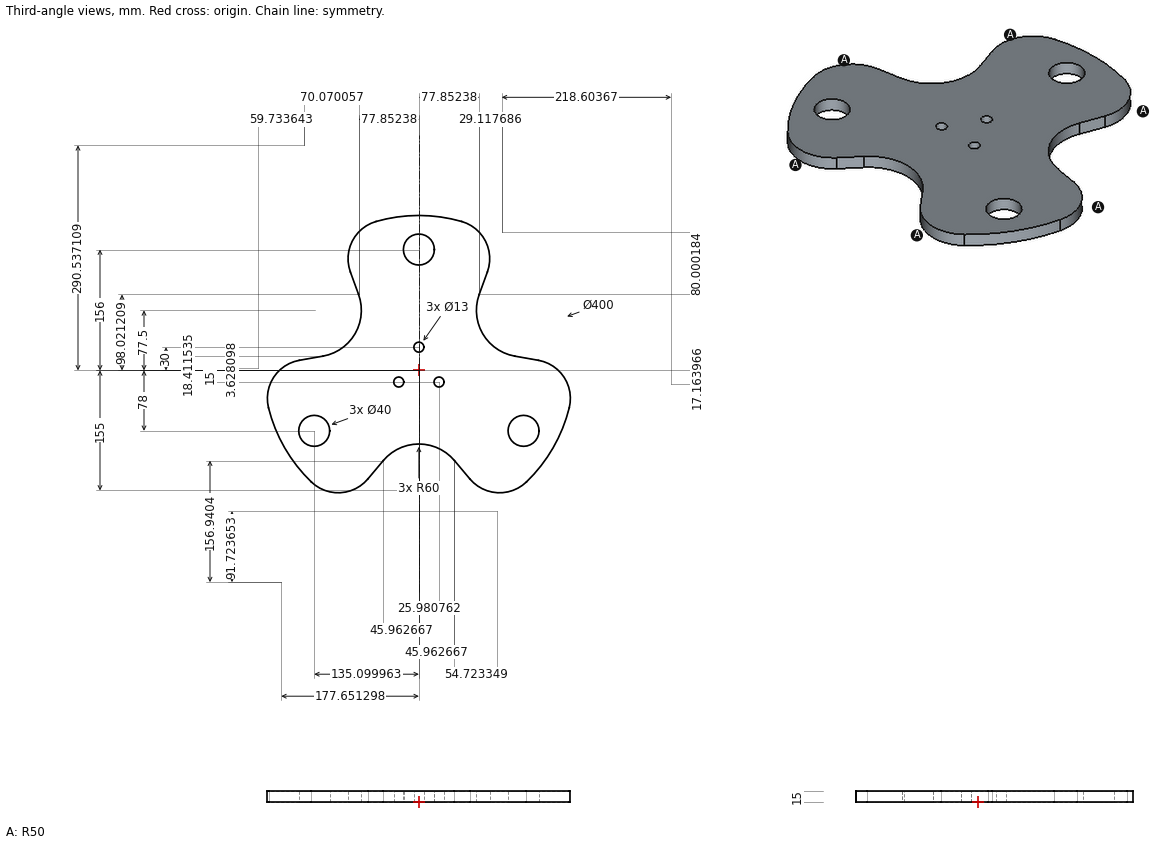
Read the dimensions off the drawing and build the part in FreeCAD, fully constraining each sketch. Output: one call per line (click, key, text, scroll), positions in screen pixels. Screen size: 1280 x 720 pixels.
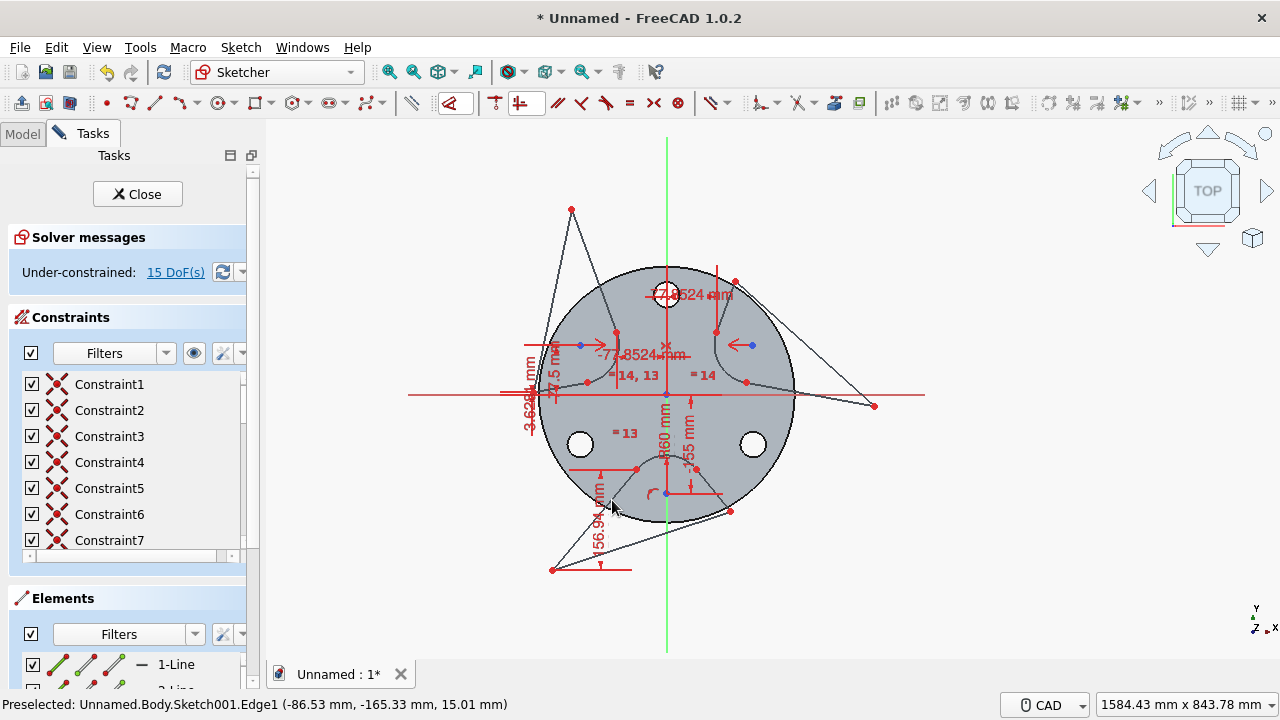
scroll(637, 470, up, 2)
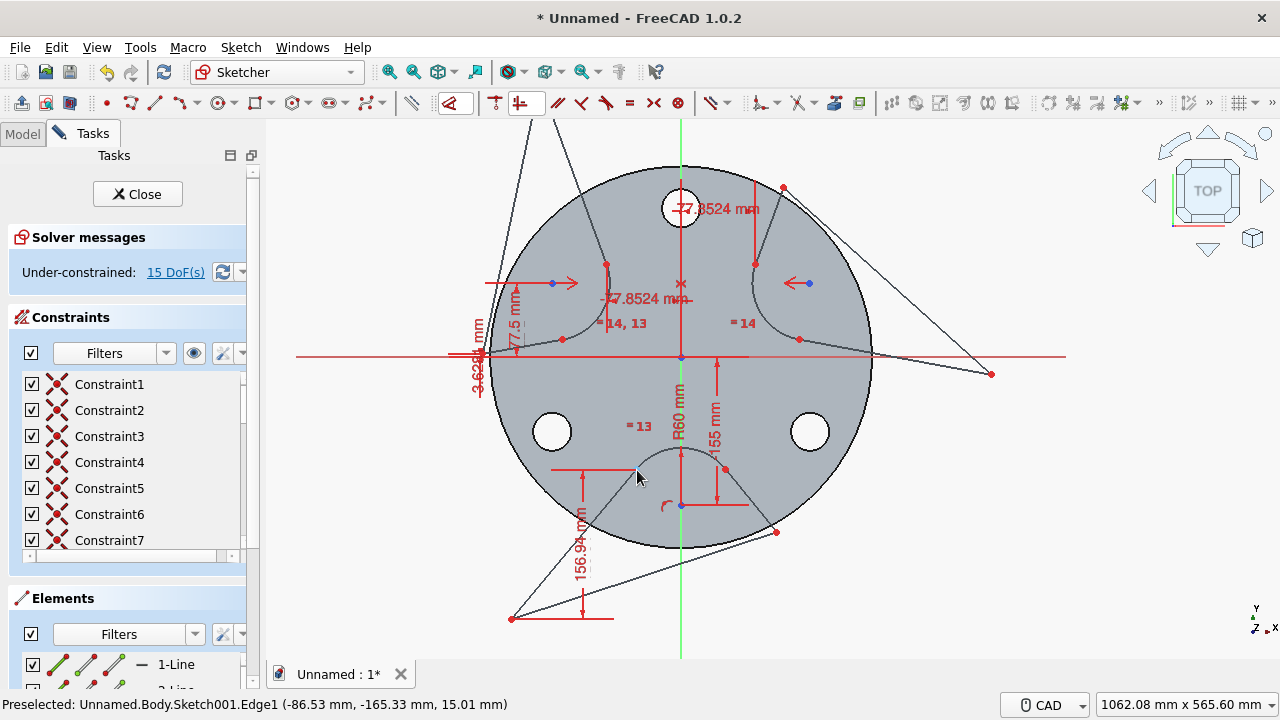
click(636, 470)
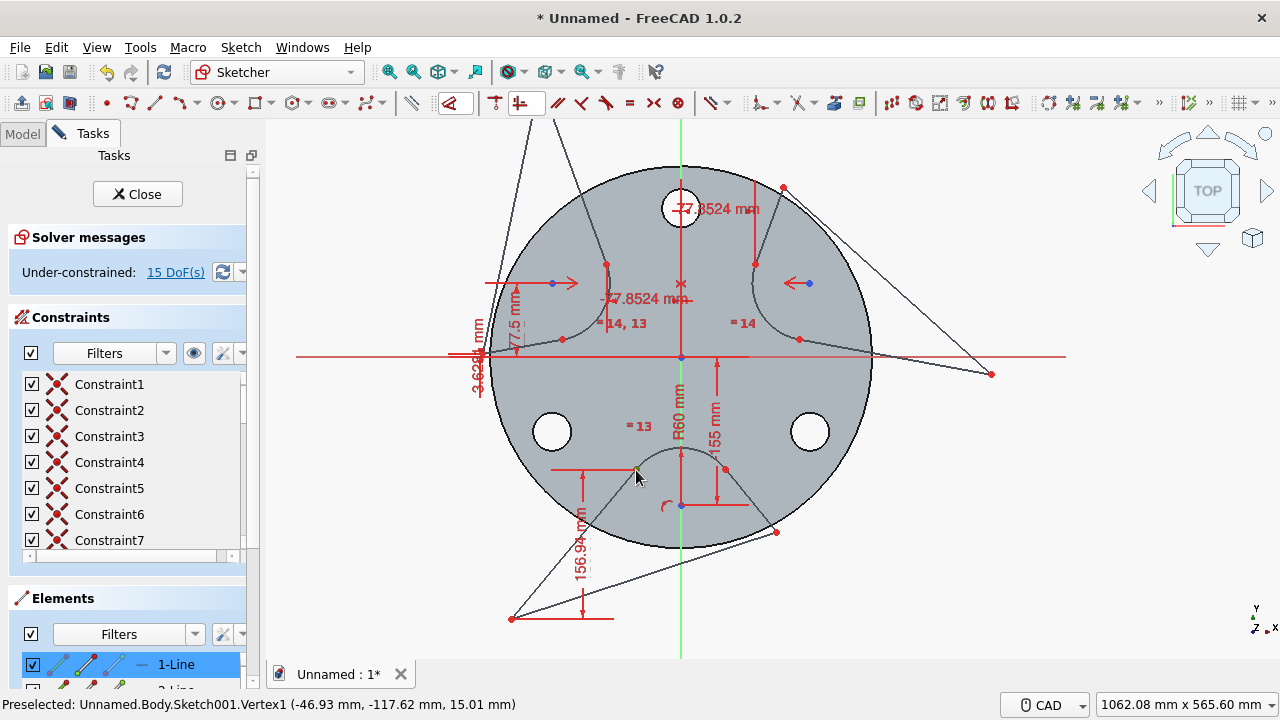
click(468, 104)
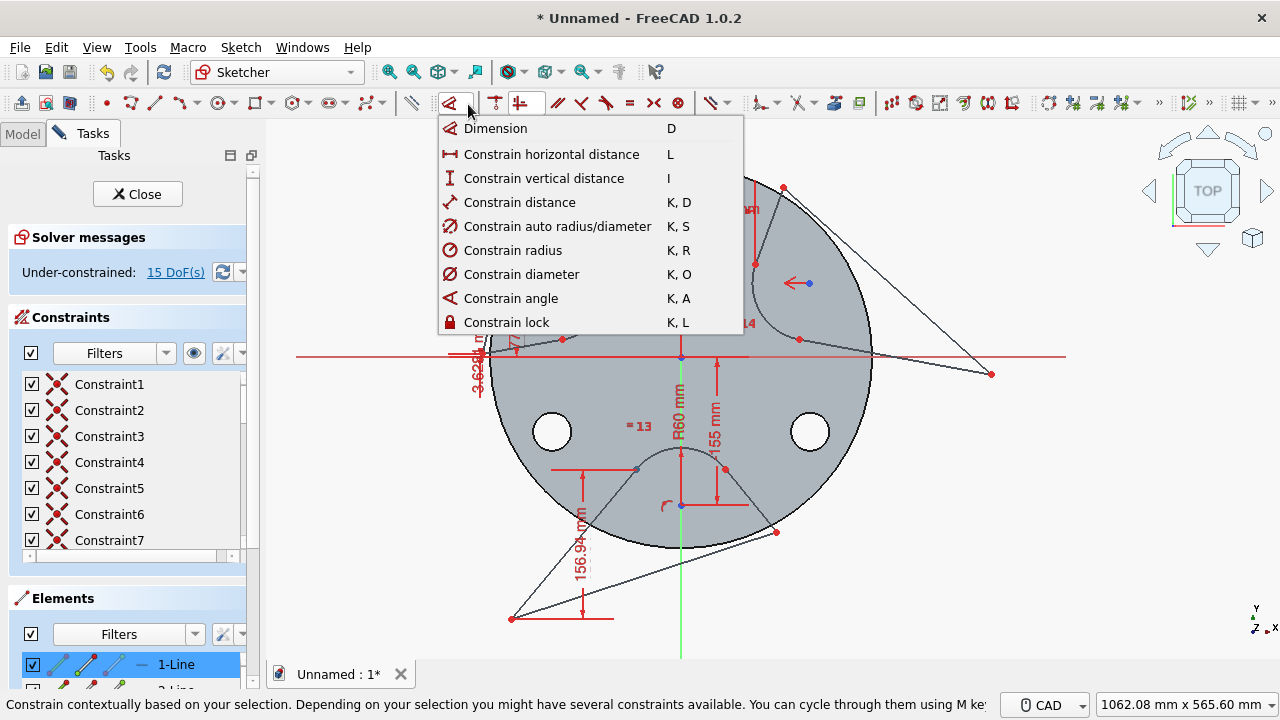
click(591, 154)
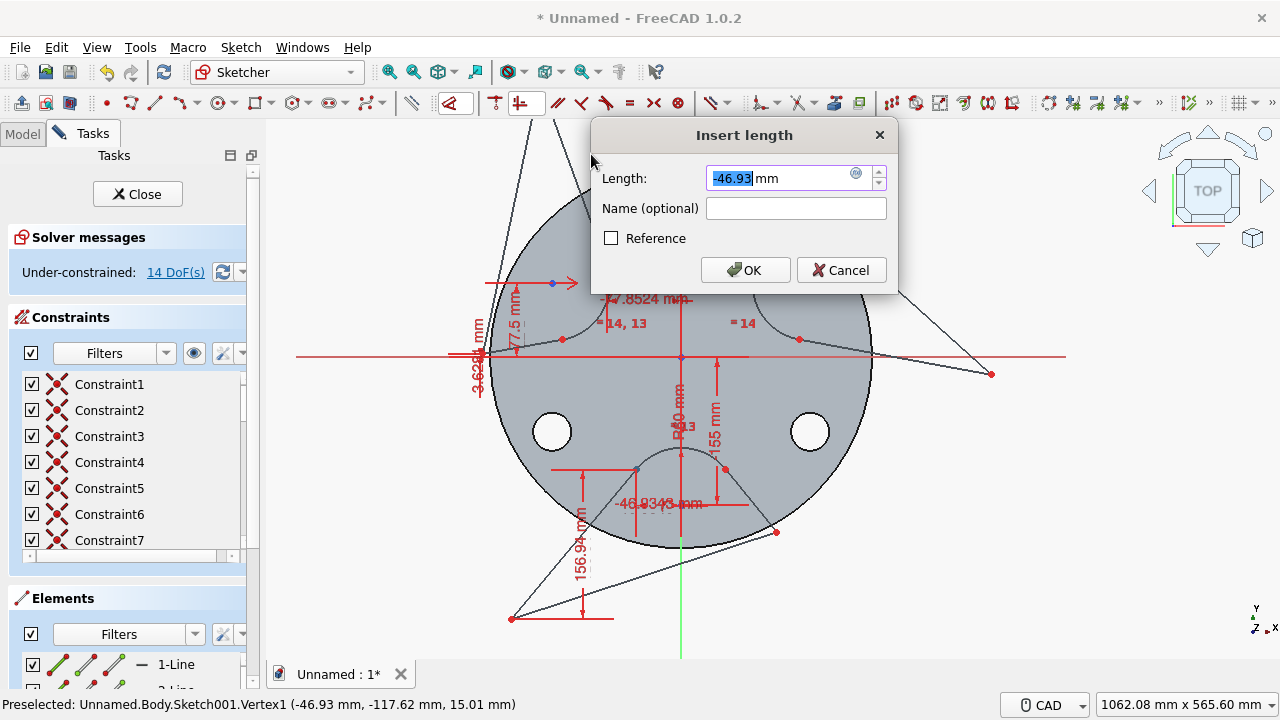
text(-45.962667)
key(Return)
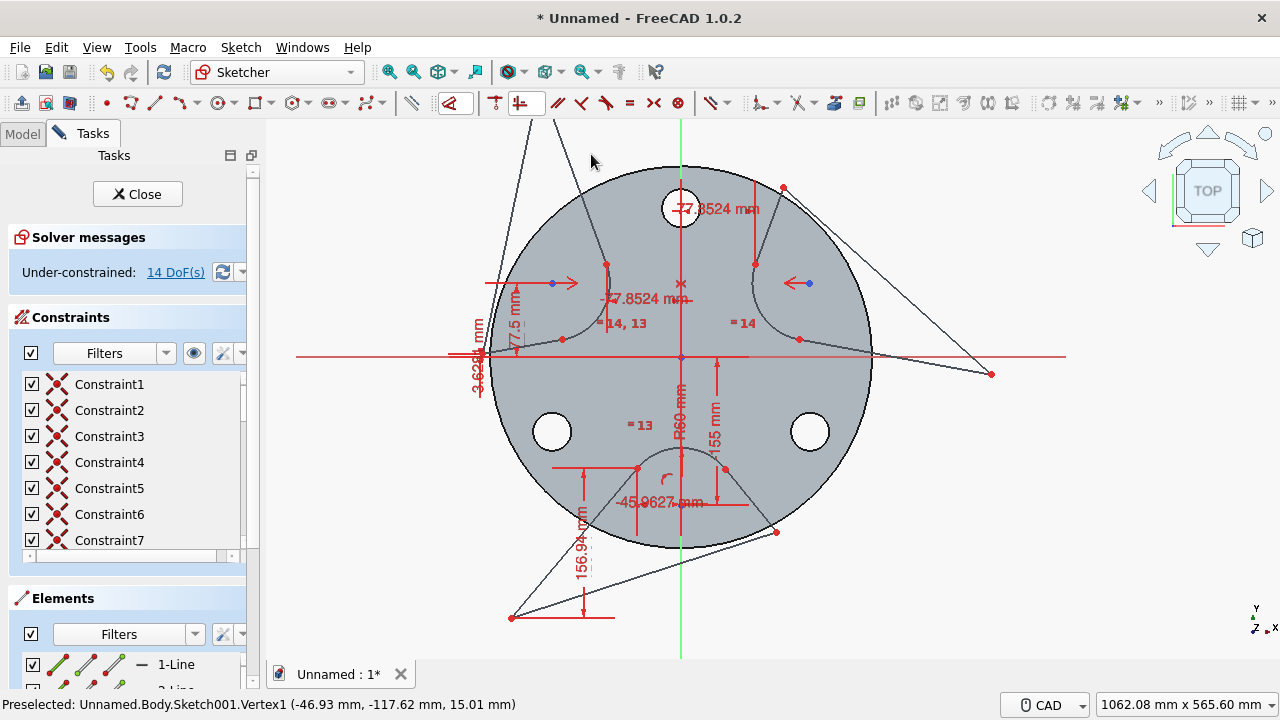
click(726, 469)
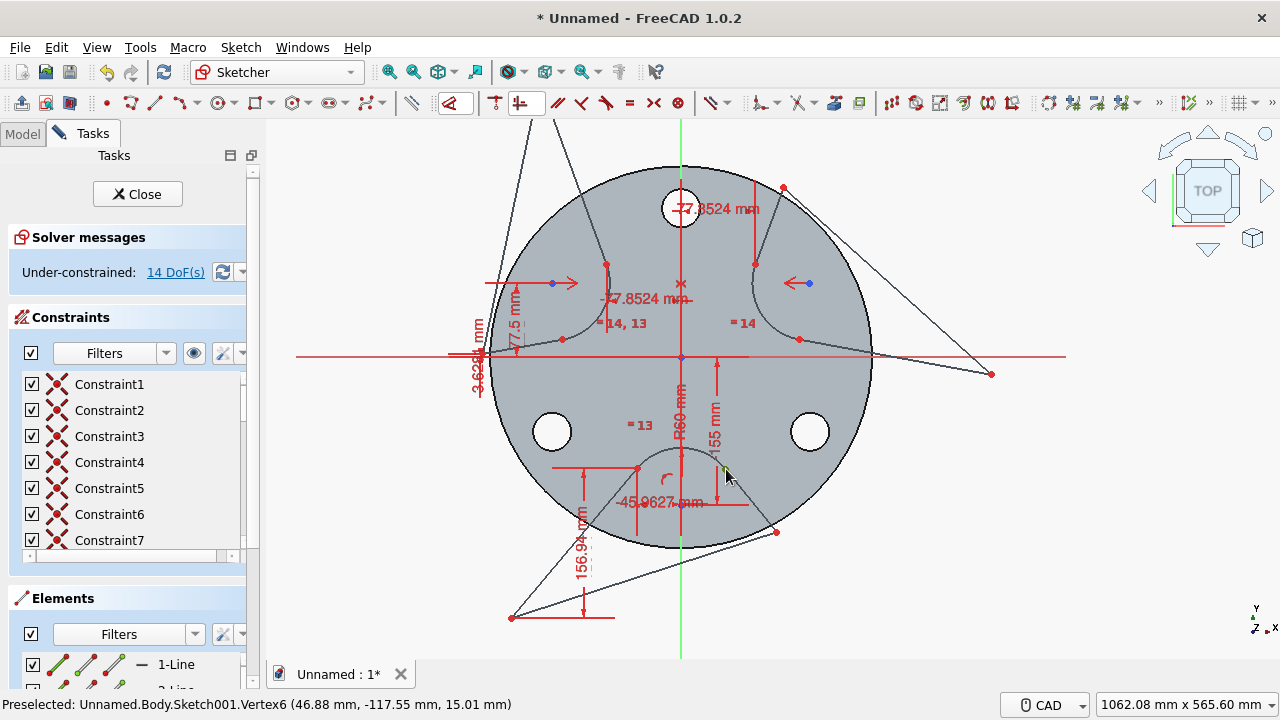
click(468, 104)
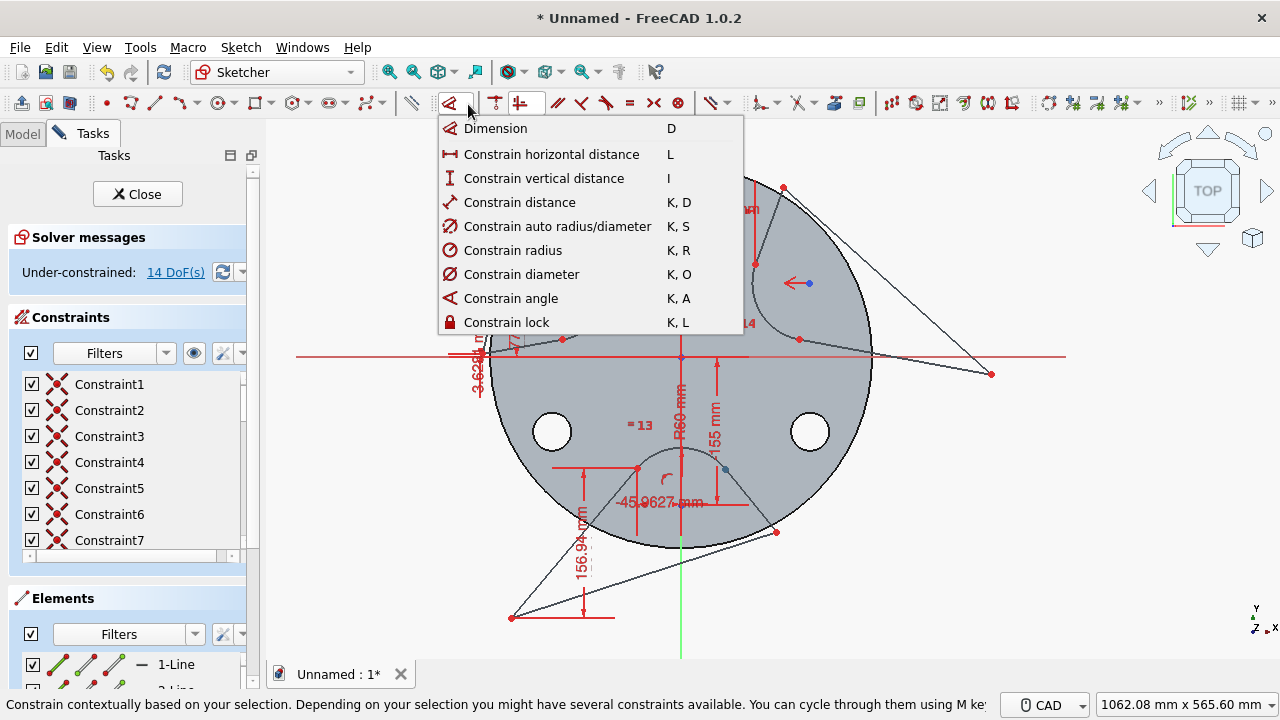
click(591, 154)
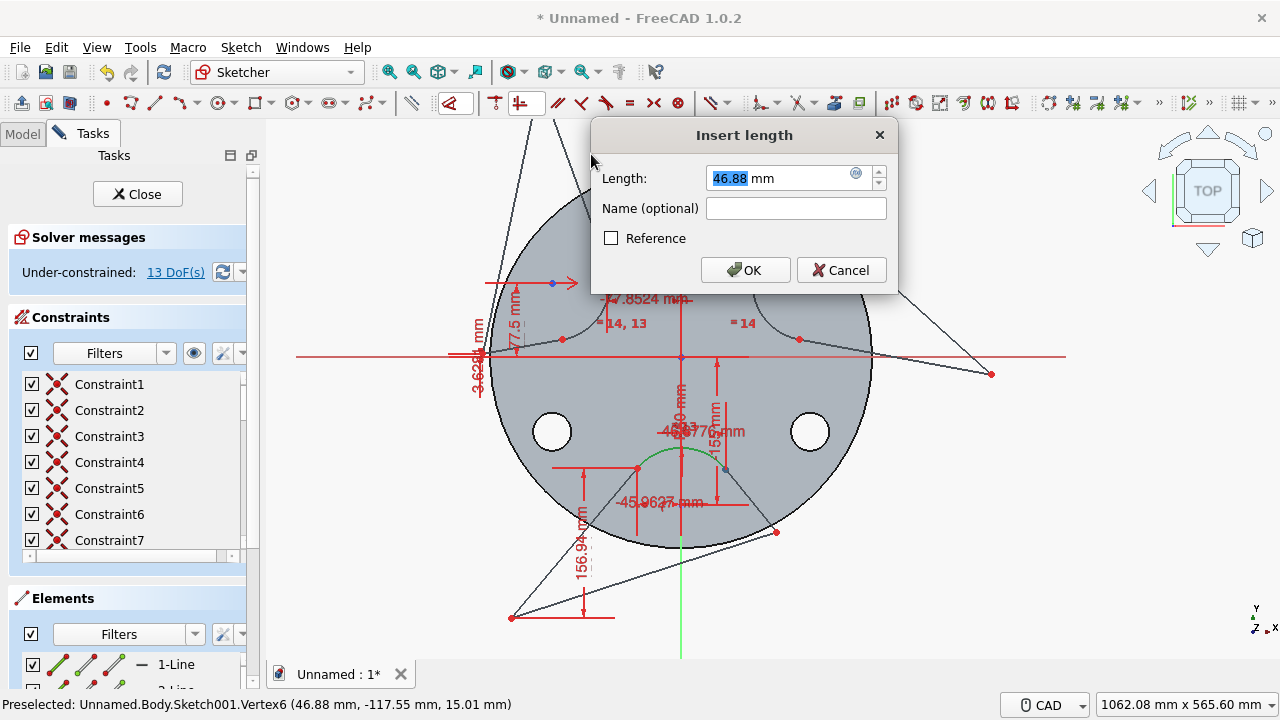
text(45.962667)
key(Return)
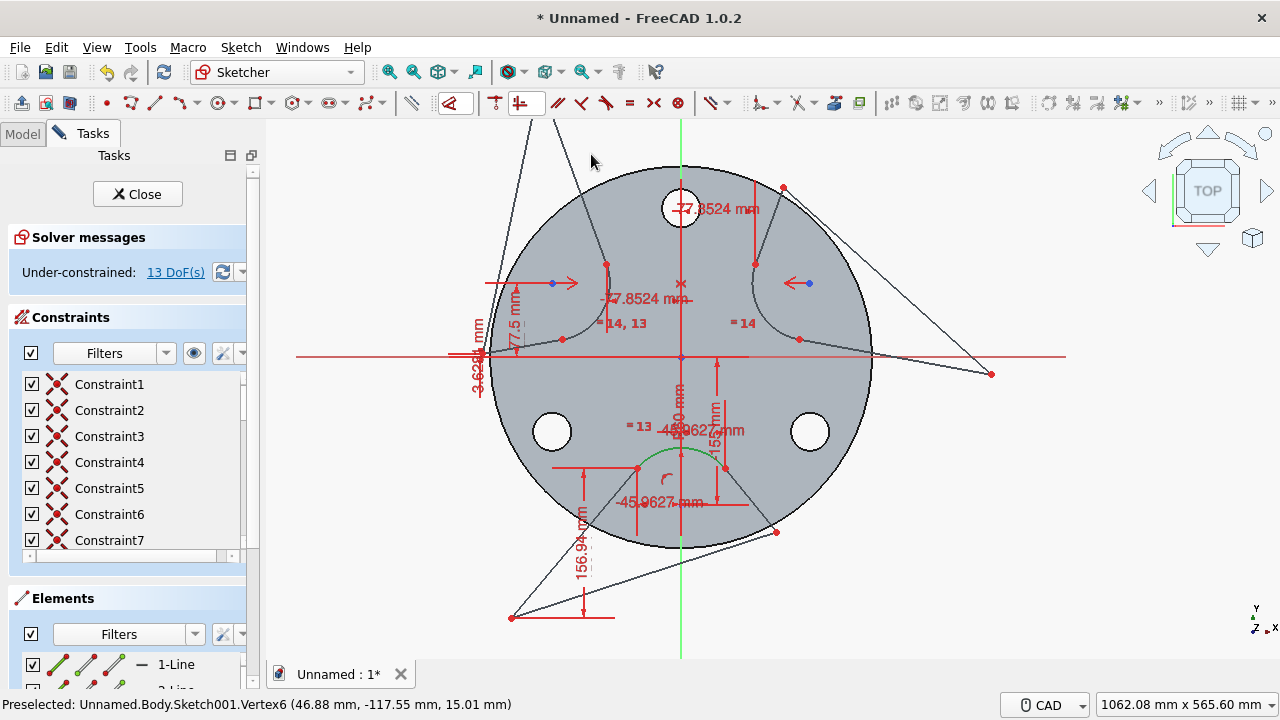
click(607, 265)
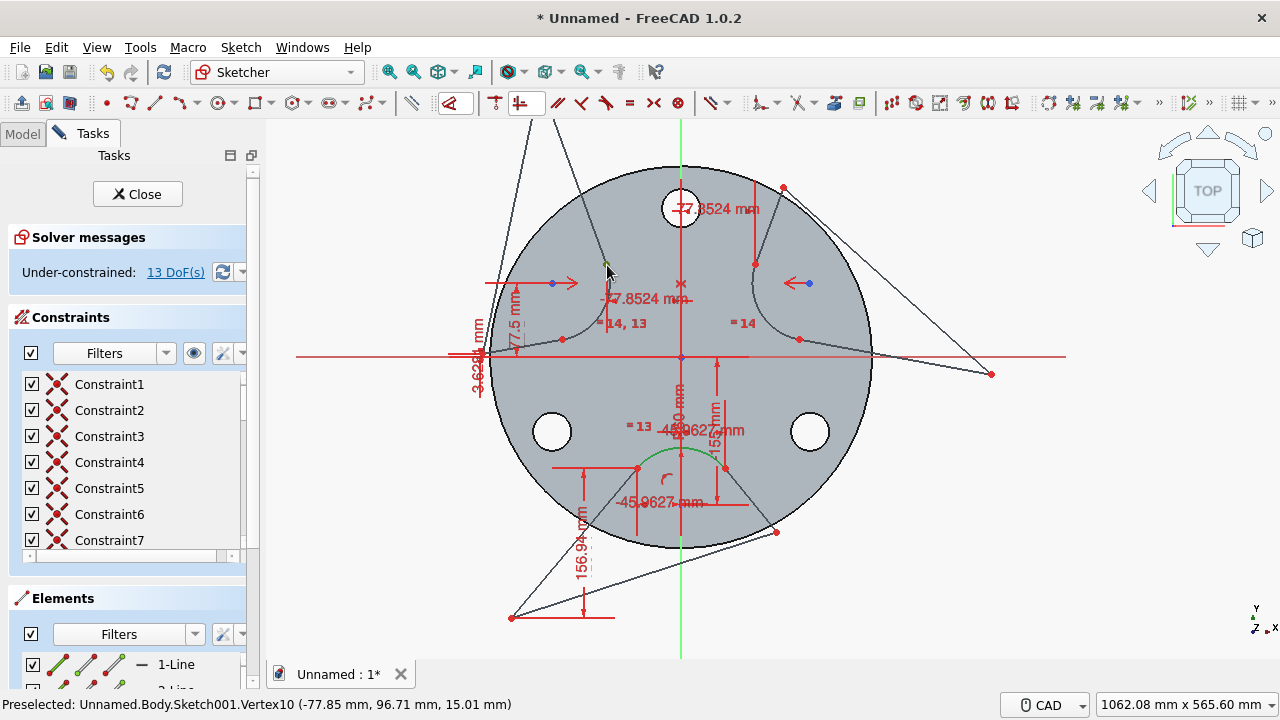
click(468, 104)